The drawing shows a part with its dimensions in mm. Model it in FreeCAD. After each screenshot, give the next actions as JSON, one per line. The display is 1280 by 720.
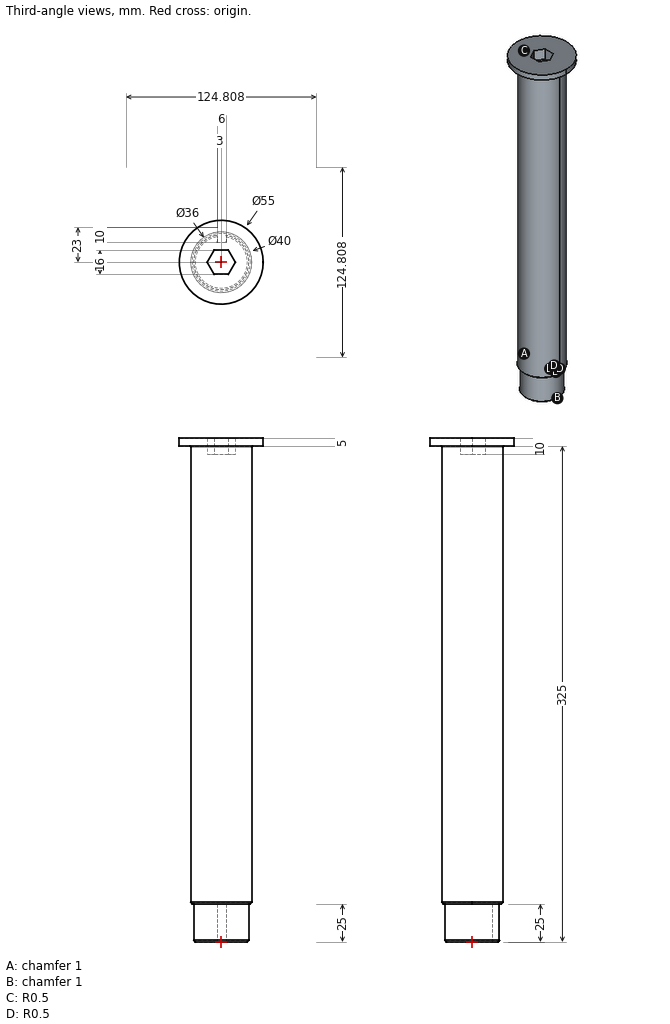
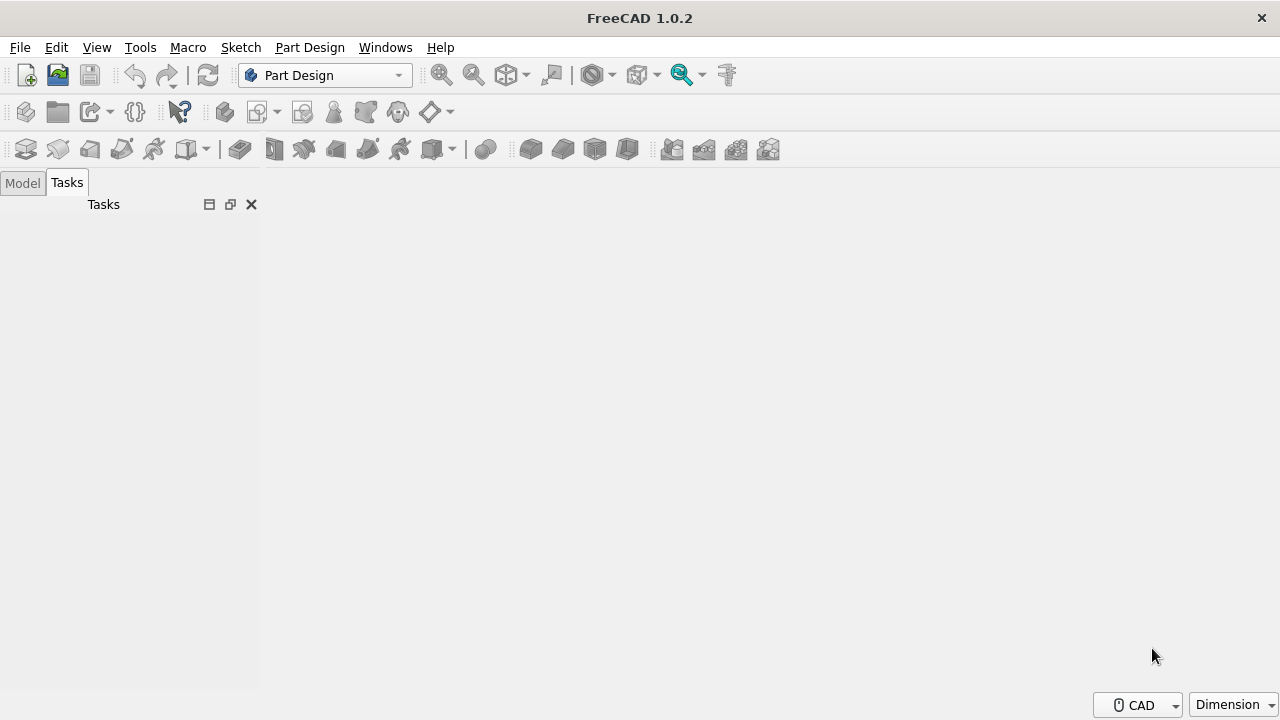
{"action": "left_click", "coordinate": [792, 76]}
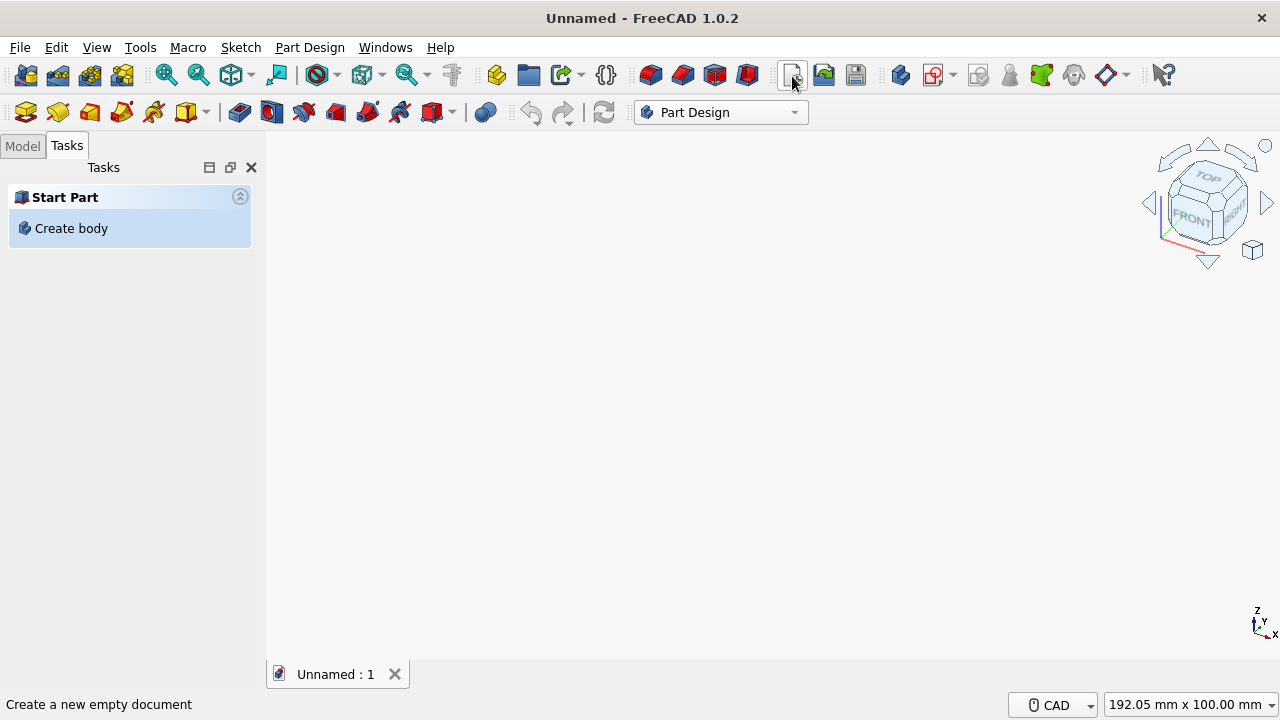
{"action": "left_click", "coordinate": [934, 76]}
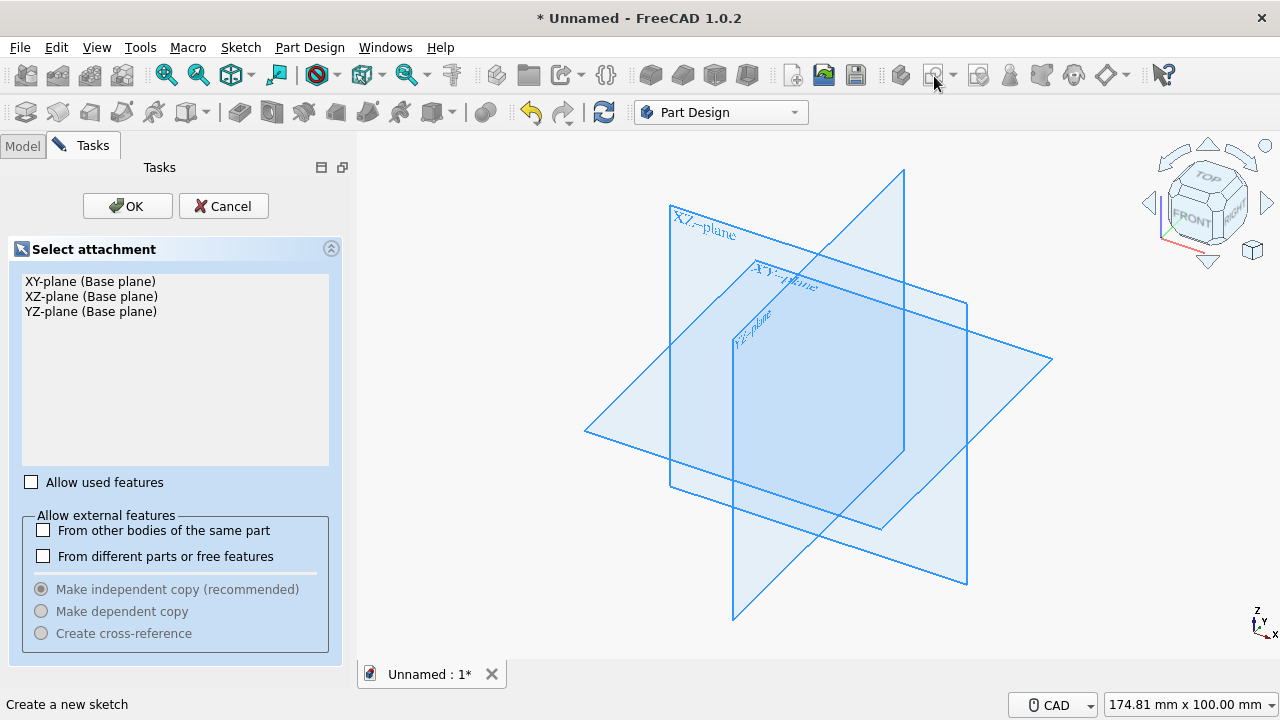
{"action": "left_click", "coordinate": [82, 282]}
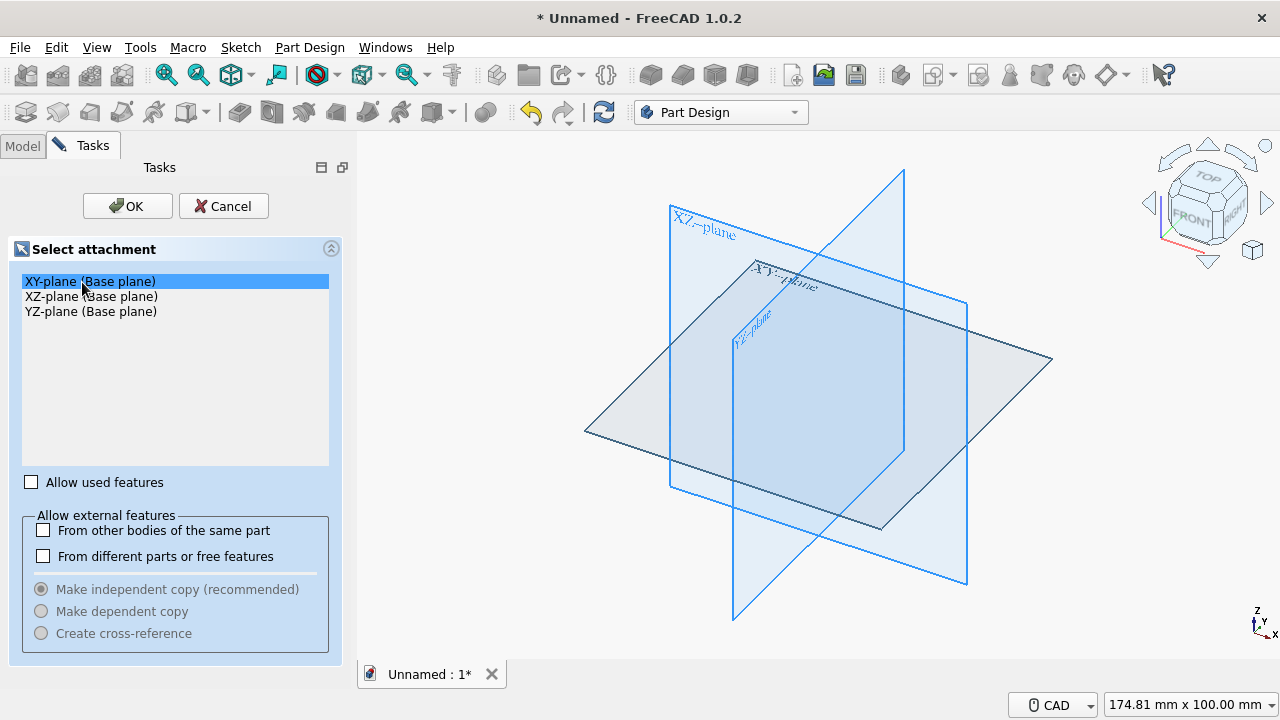
{"action": "left_click", "coordinate": [128, 206]}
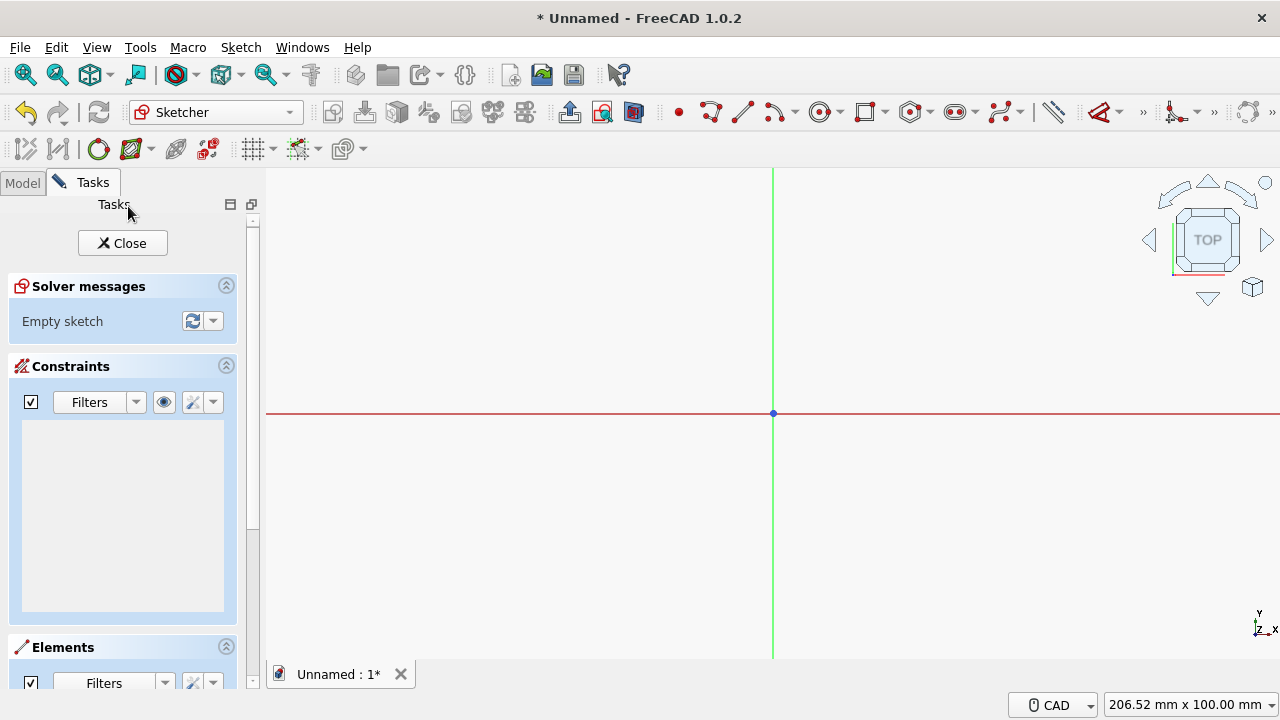
{"action": "scroll", "coordinate": [912, 413], "scroll_direction": "up", "scroll_amount": 2}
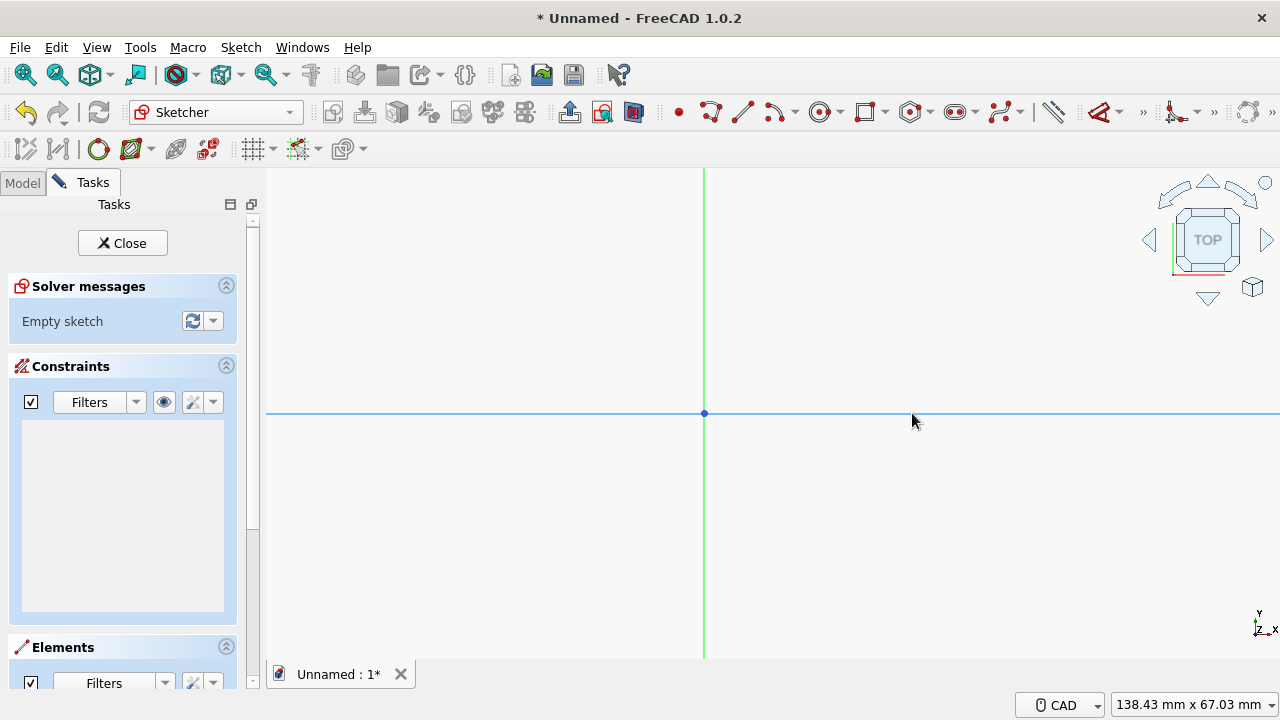
{"action": "left_click", "coordinate": [820, 112]}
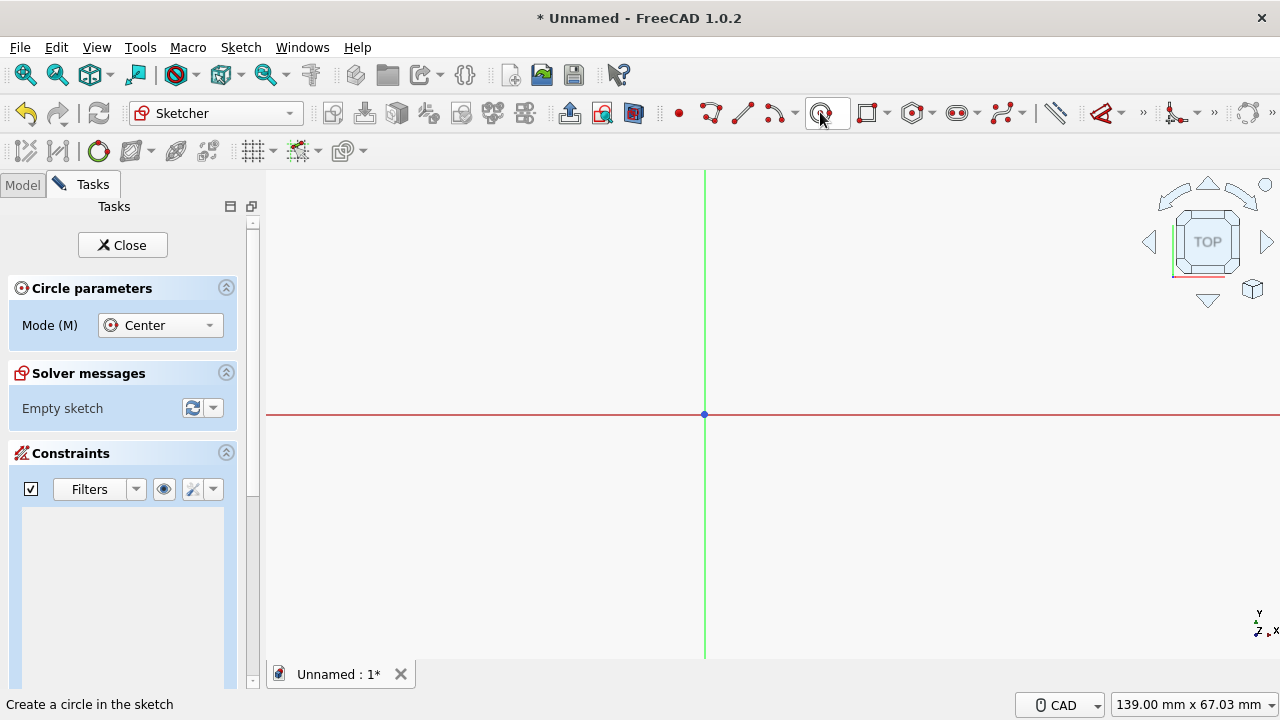
{"action": "left_click", "coordinate": [705, 414]}
{"action": "left_click", "coordinate": [808, 311]}
{"action": "key", "text": "Escape"}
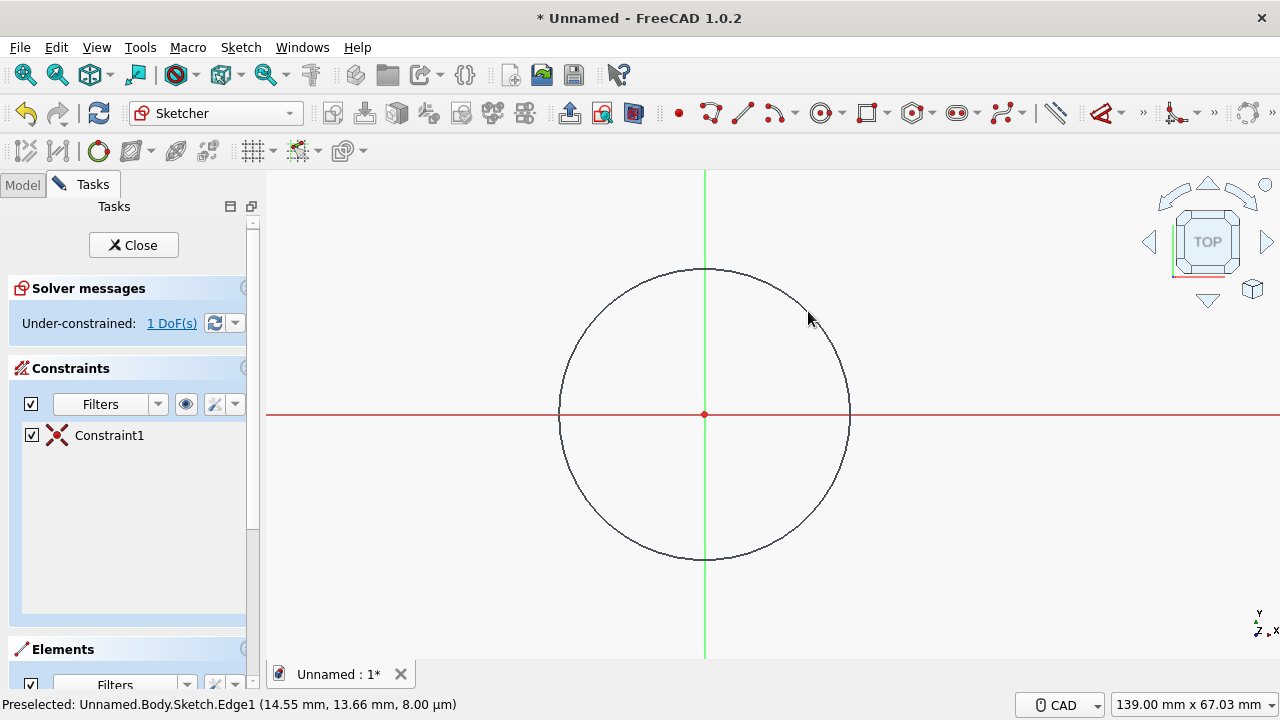
{"action": "left_click", "coordinate": [1102, 114]}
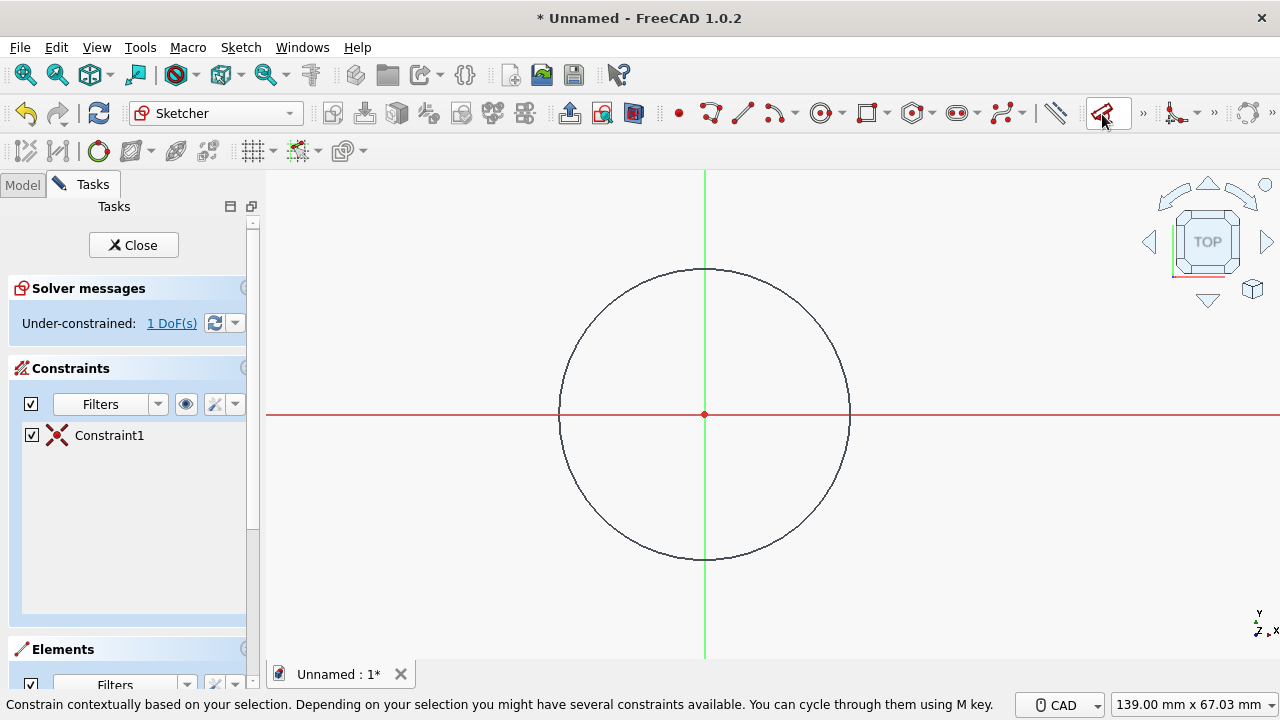
{"action": "left_click", "coordinate": [807, 311]}
{"action": "left_click", "coordinate": [830, 288]}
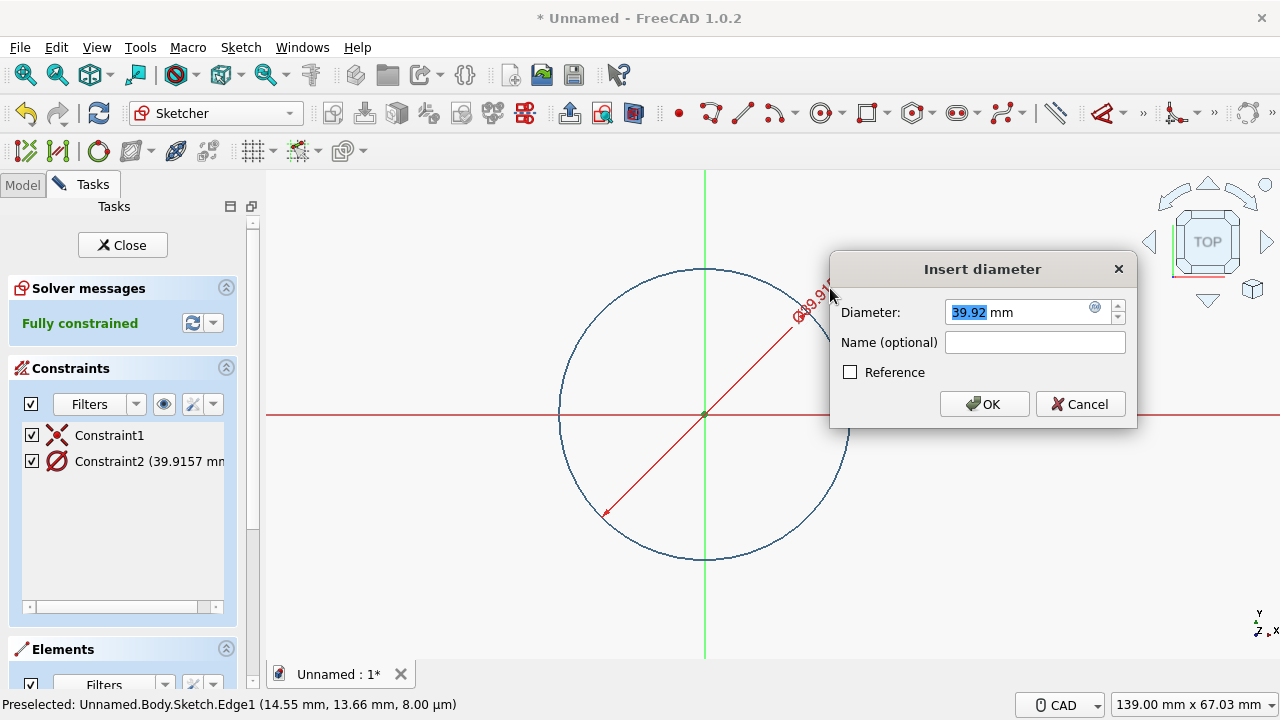
{"action": "type", "text": "40"}
{"action": "key", "text": "Return"}
{"action": "key", "text": "Escape"}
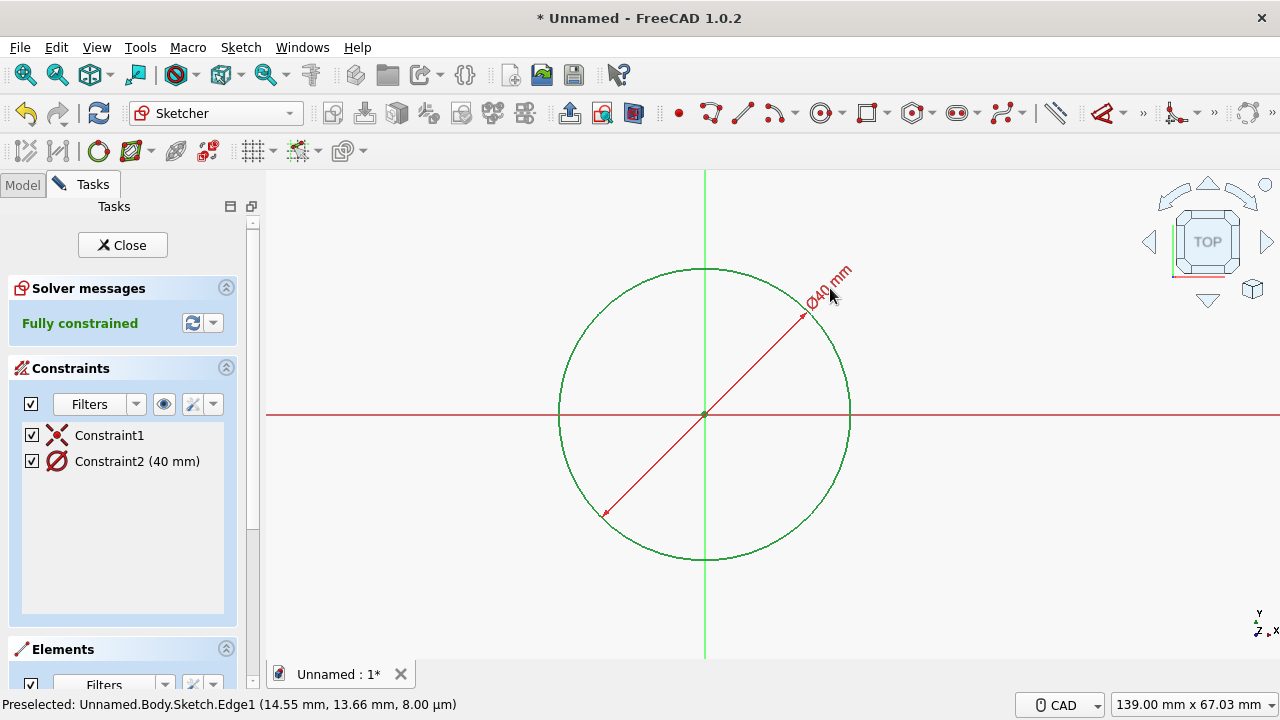
{"action": "left_click", "coordinate": [123, 245]}